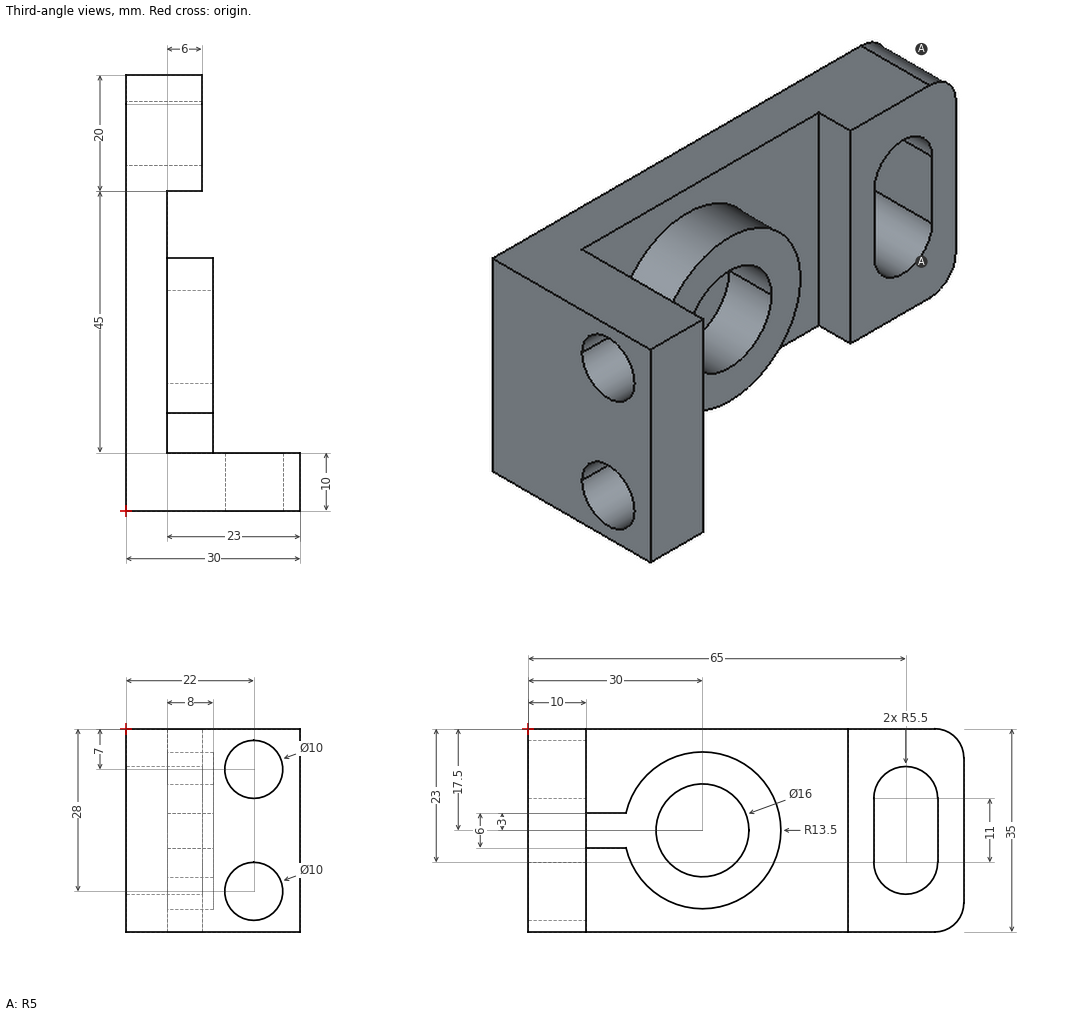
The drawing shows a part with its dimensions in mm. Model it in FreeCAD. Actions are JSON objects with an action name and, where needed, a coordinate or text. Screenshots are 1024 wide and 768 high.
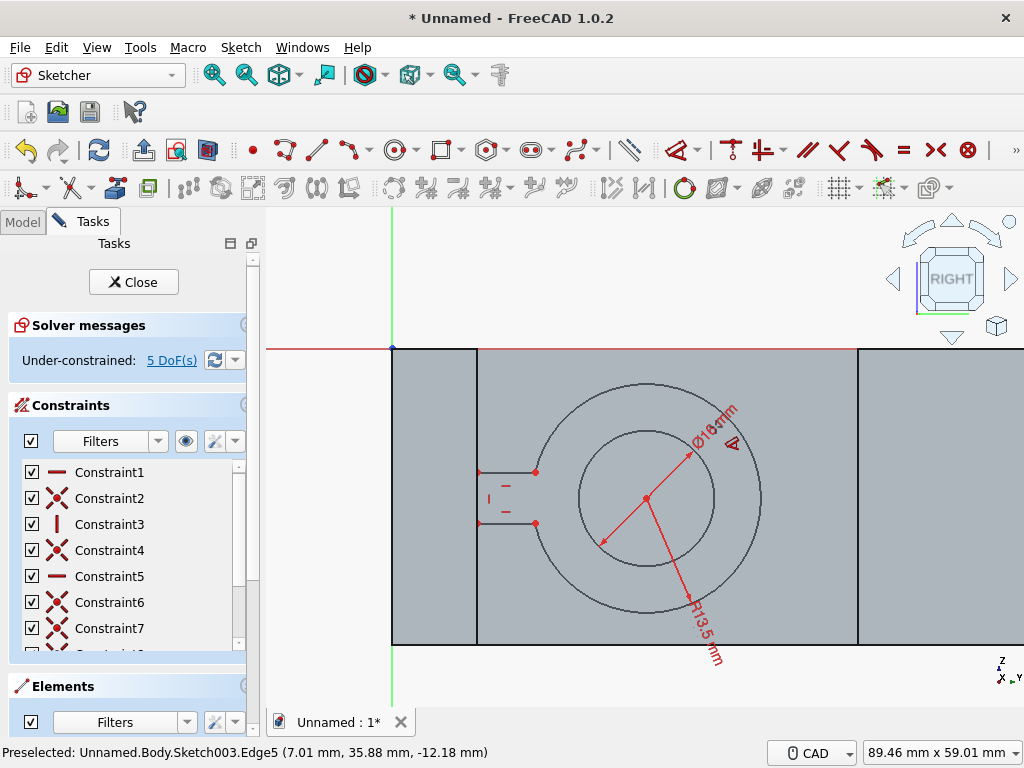
{"action": "left_click", "coordinate": [477, 488]}
{"action": "left_click", "coordinate": [443, 499]}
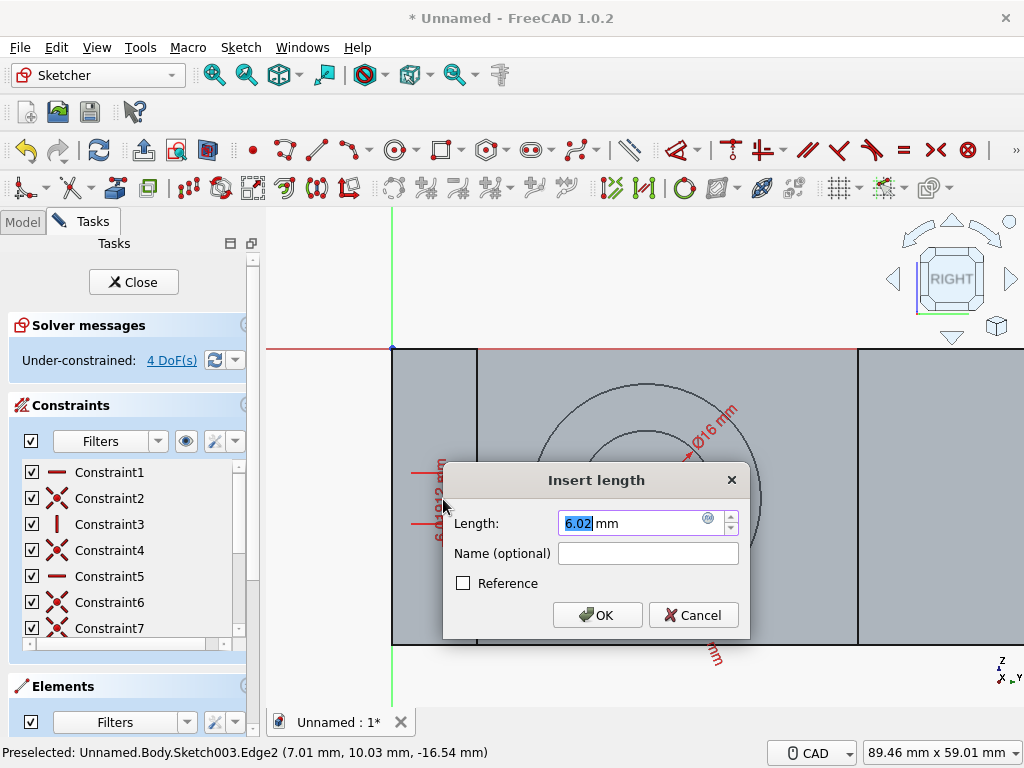
{"action": "type", "text": "6"}
{"action": "key", "text": "Return"}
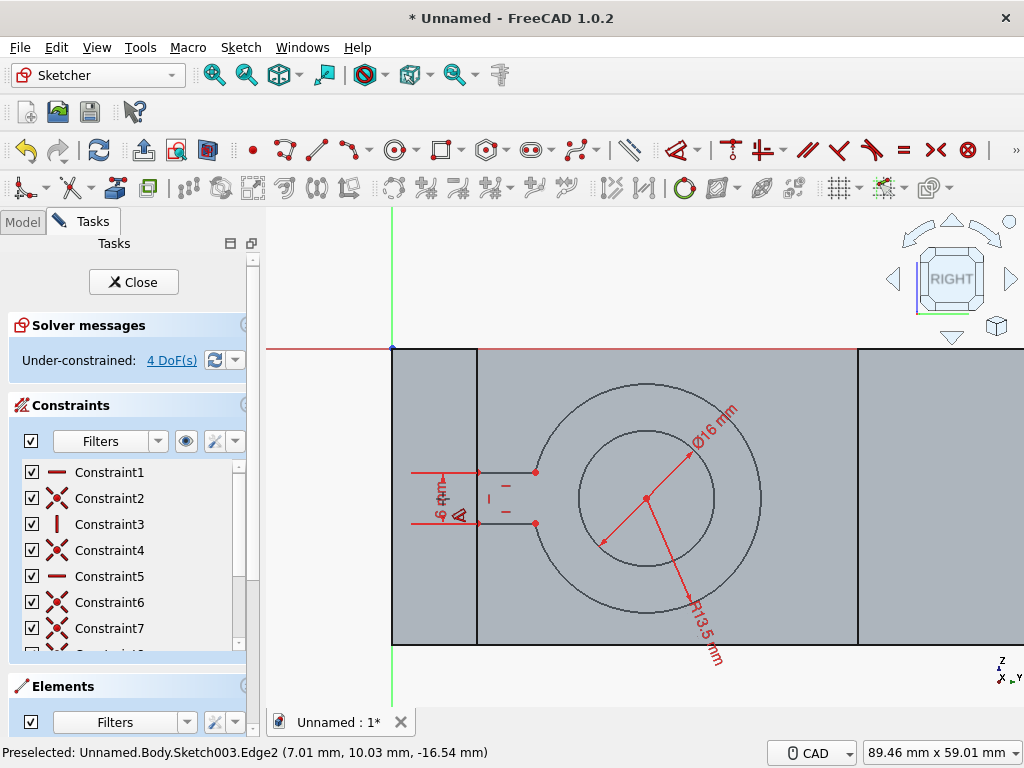
{"action": "left_click", "coordinate": [647, 498]}
{"action": "left_click", "coordinate": [519, 315]}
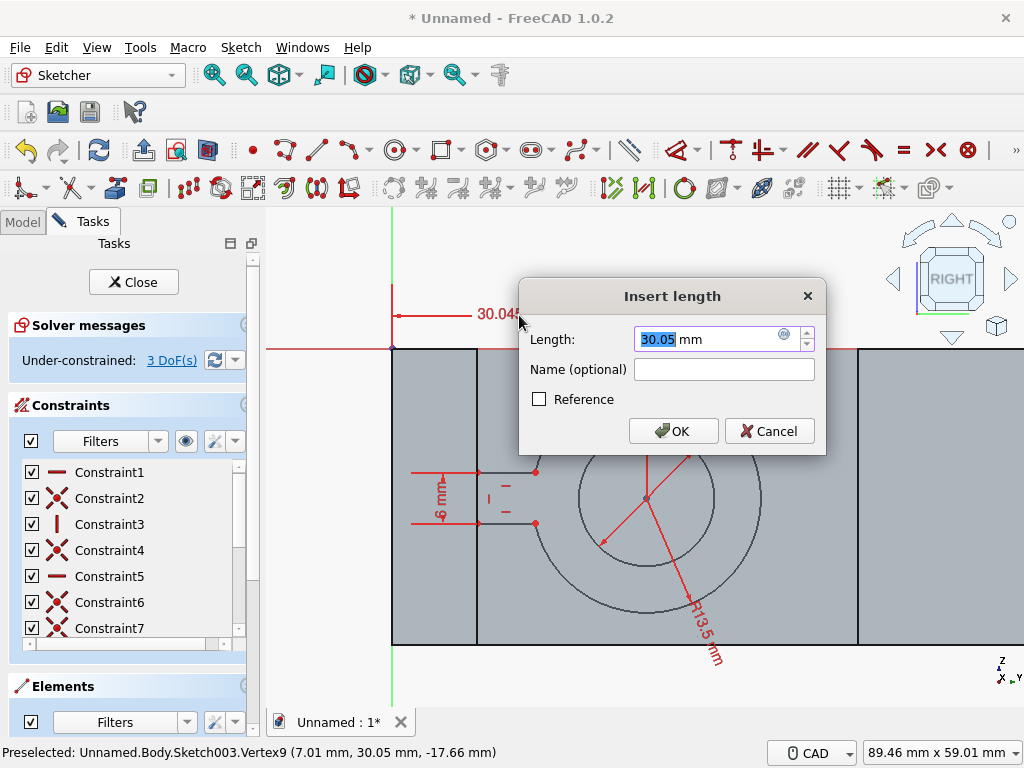
{"action": "type", "text": "30"}
{"action": "key", "text": "Return"}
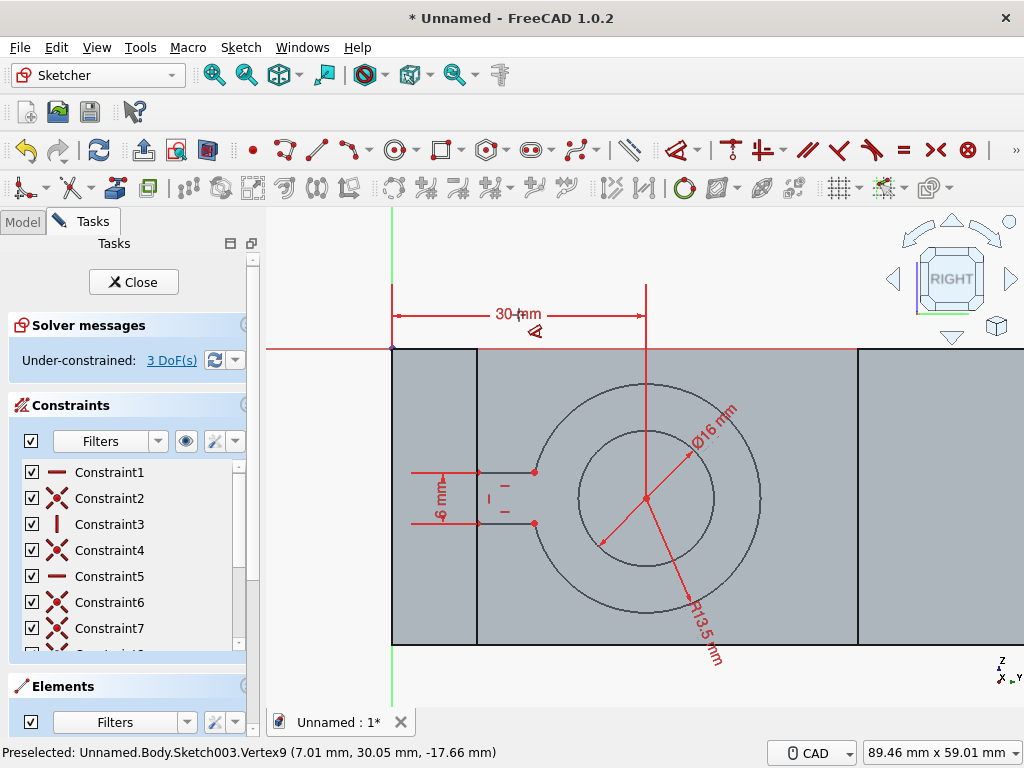
{"action": "scroll", "coordinate": [535, 473], "scroll_direction": "up", "scroll_amount": 3}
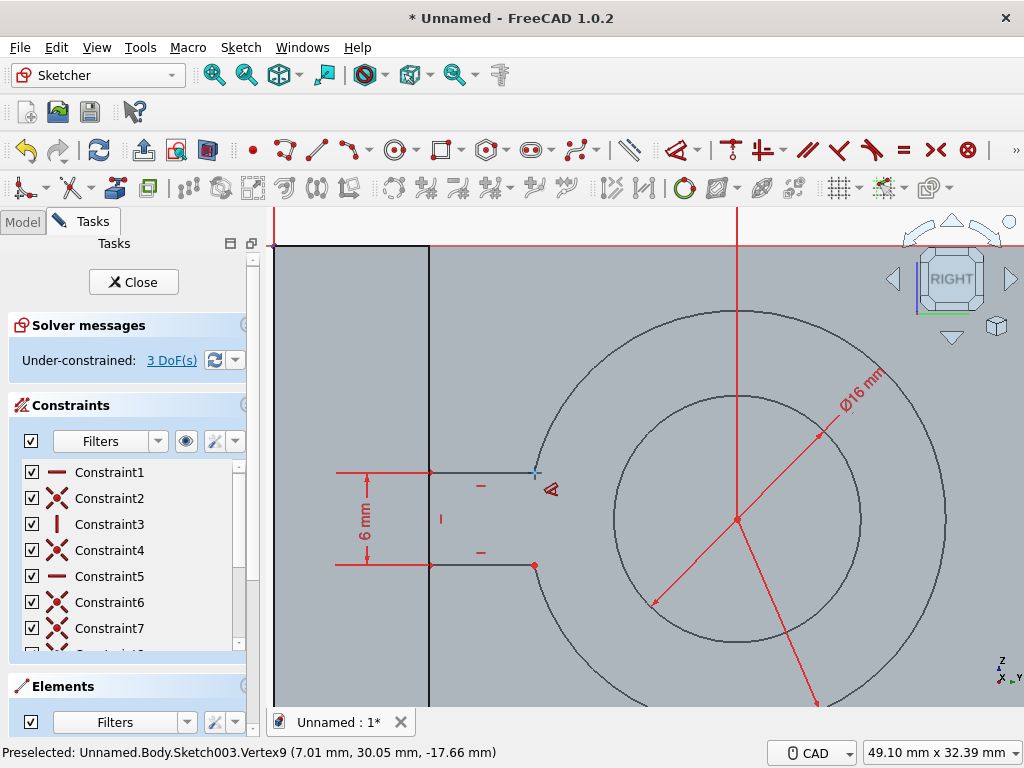
{"action": "left_click", "coordinate": [534, 473]}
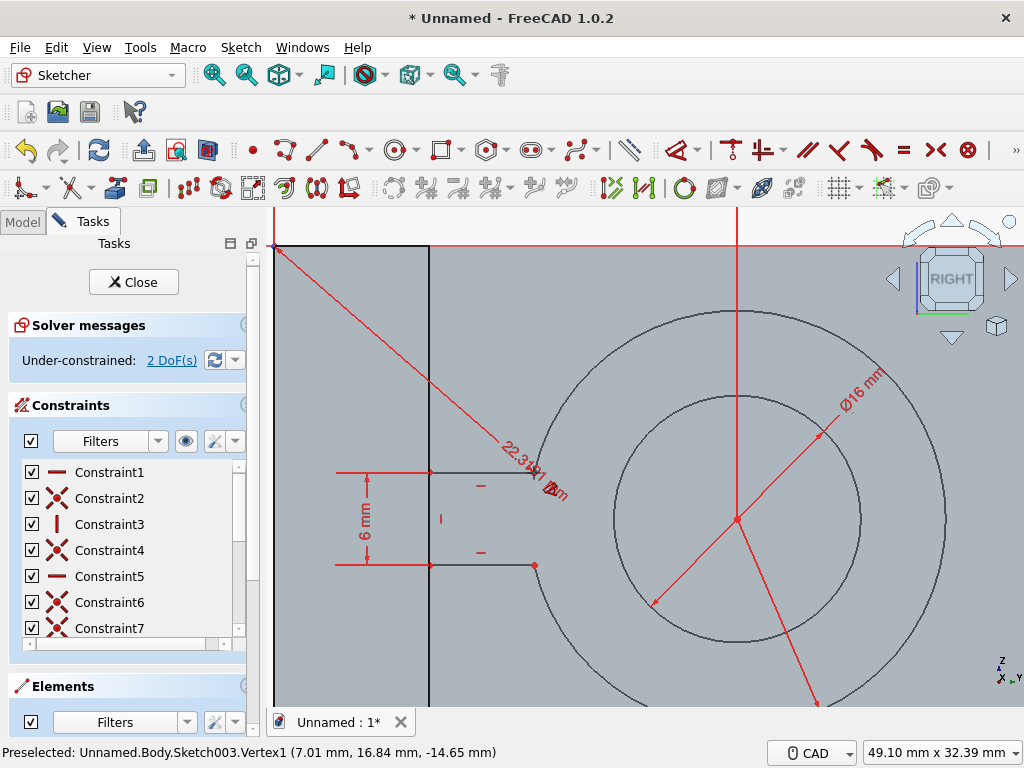
{"action": "left_click", "coordinate": [737, 519]}
{"action": "left_click", "coordinate": [771, 496]}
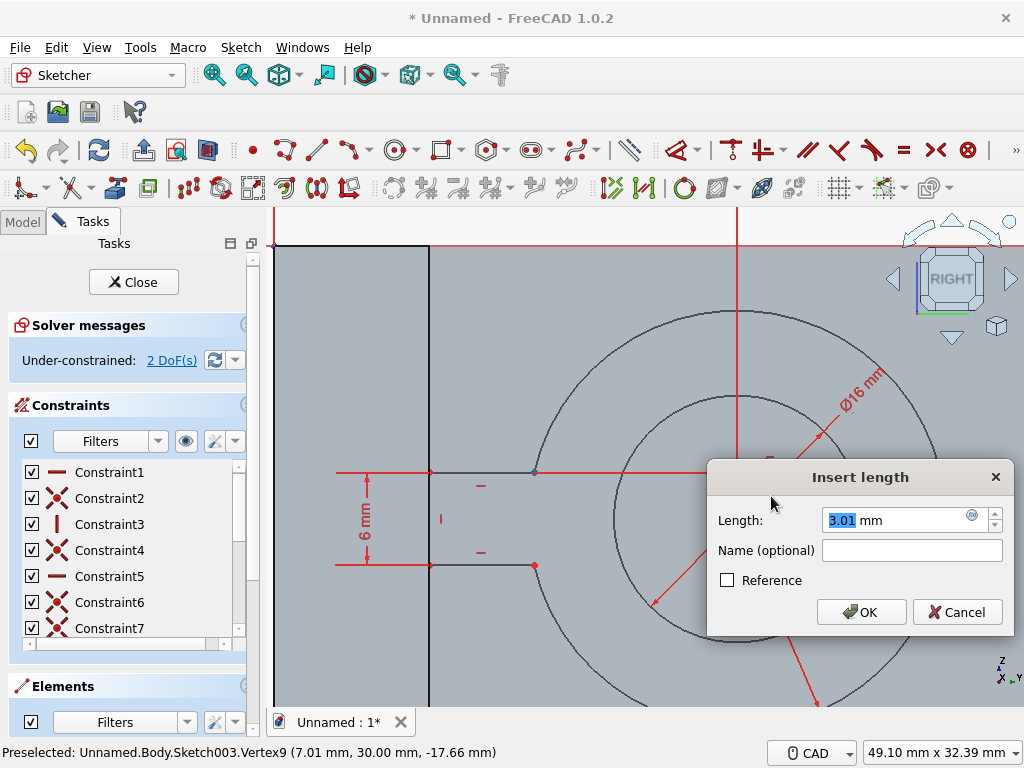
{"action": "type", "text": "3"}
{"action": "key", "text": "Return"}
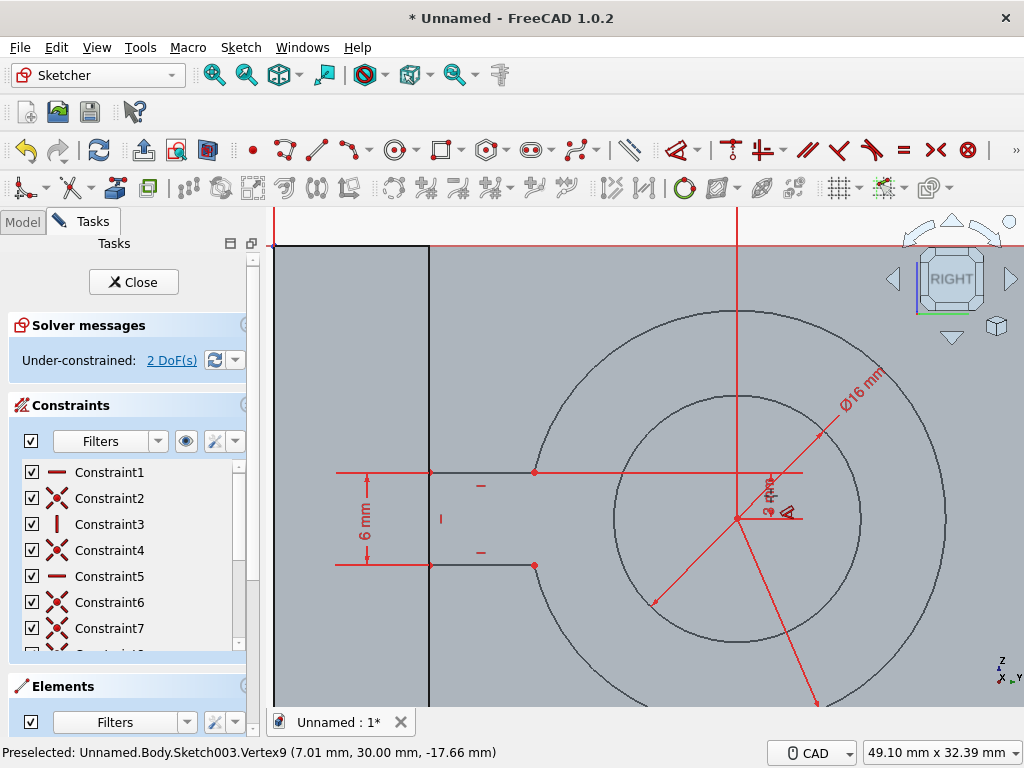
{"action": "left_click", "coordinate": [429, 473]}
{"action": "left_click", "coordinate": [362, 555]}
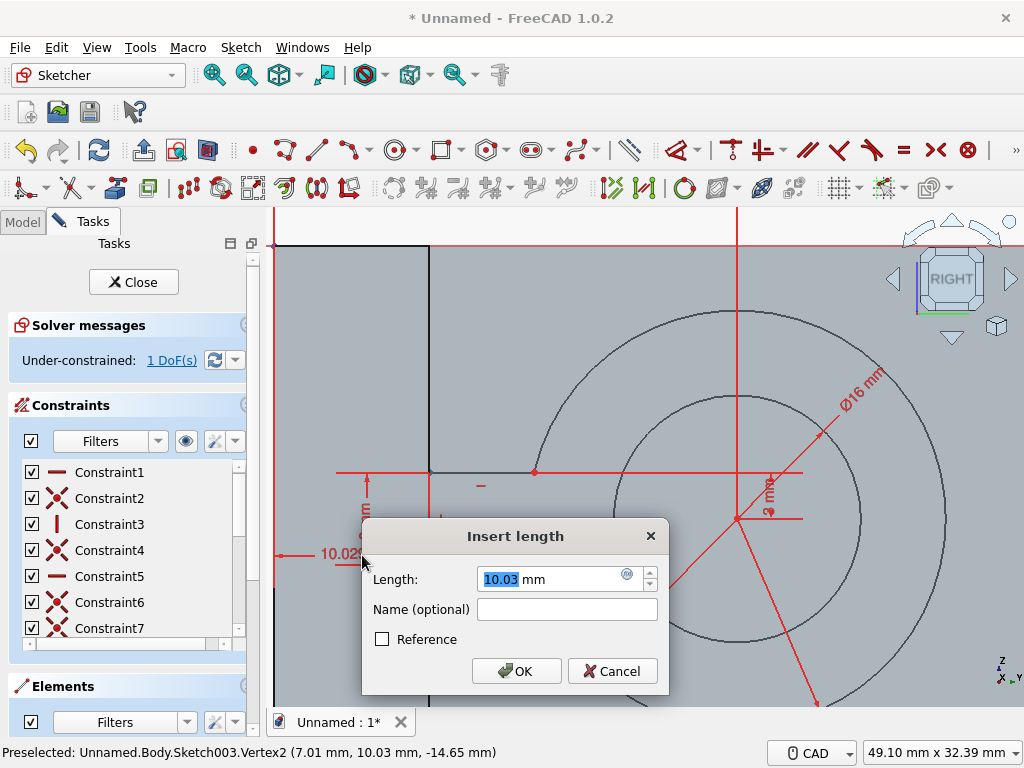
{"action": "type", "text": "10"}
{"action": "key", "text": "Return"}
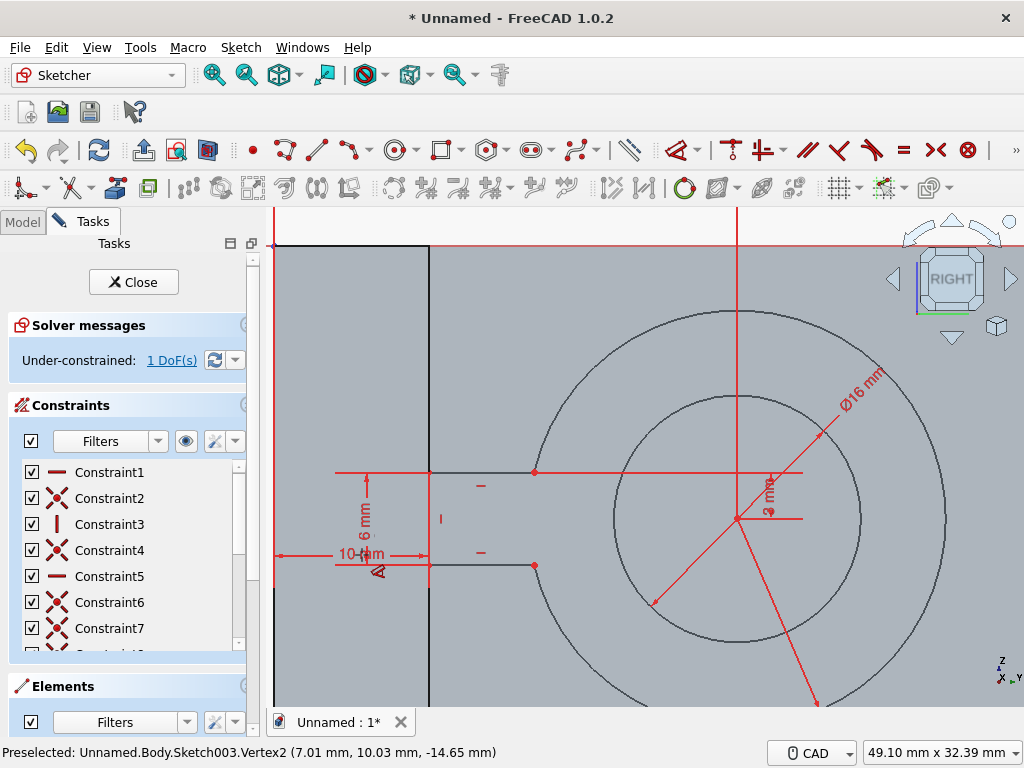
{"action": "left_click", "coordinate": [737, 519]}
{"action": "left_click", "coordinate": [771, 383]}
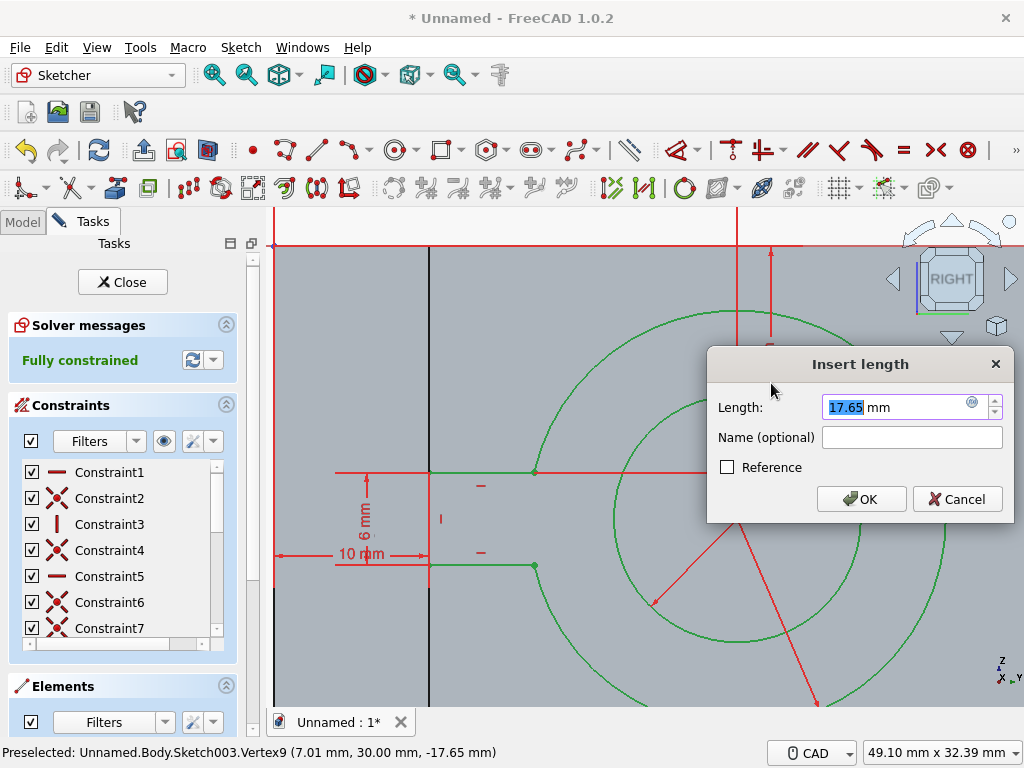
{"action": "type", "text": "17.5"}
{"action": "key", "text": "Return"}
{"action": "key", "text": "Escape"}